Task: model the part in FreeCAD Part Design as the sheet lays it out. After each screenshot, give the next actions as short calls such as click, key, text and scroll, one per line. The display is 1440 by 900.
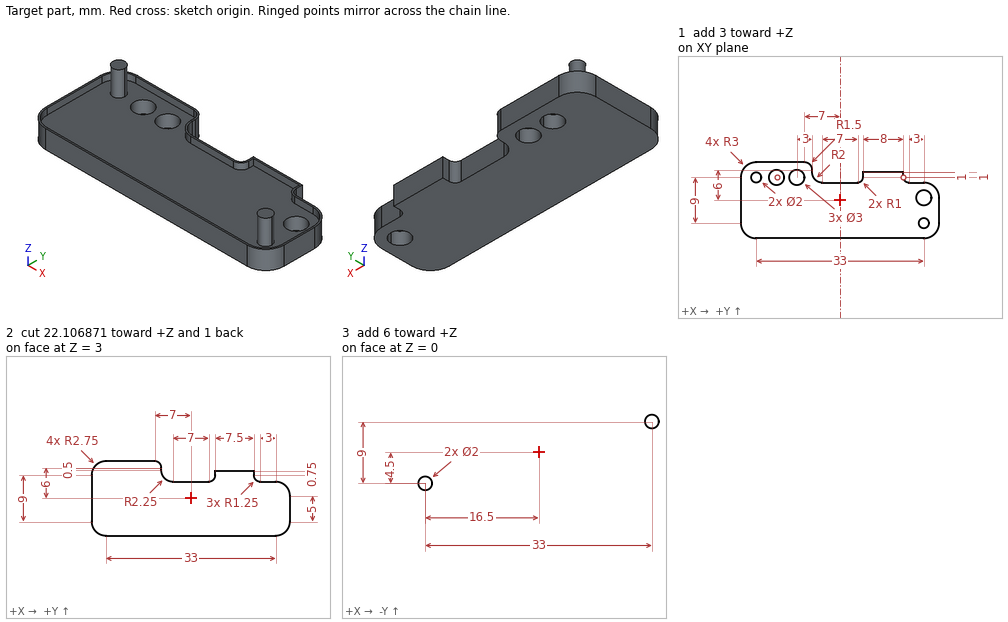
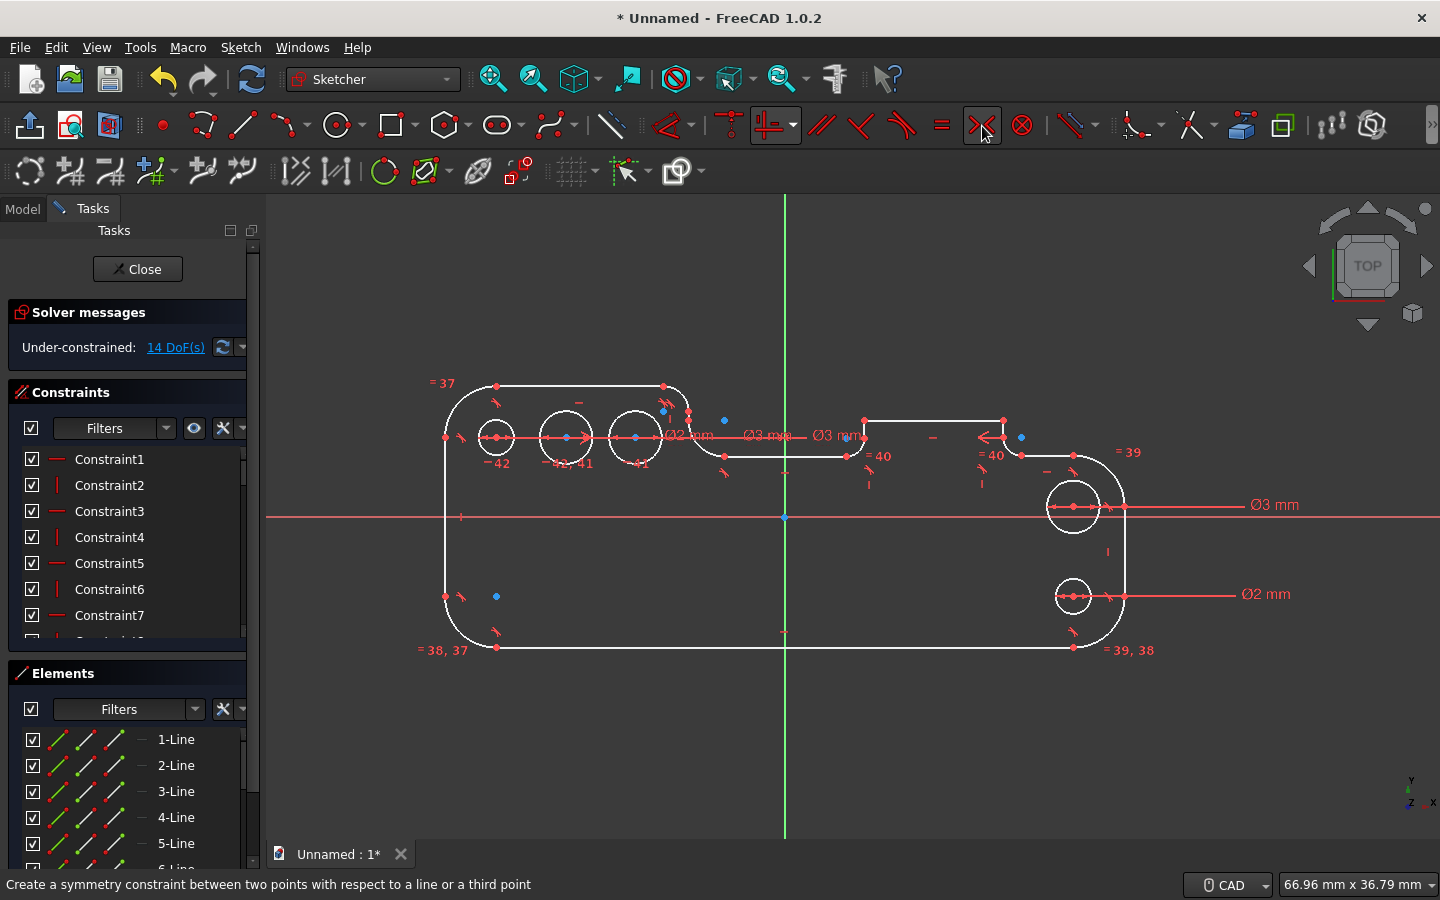
click(666, 126)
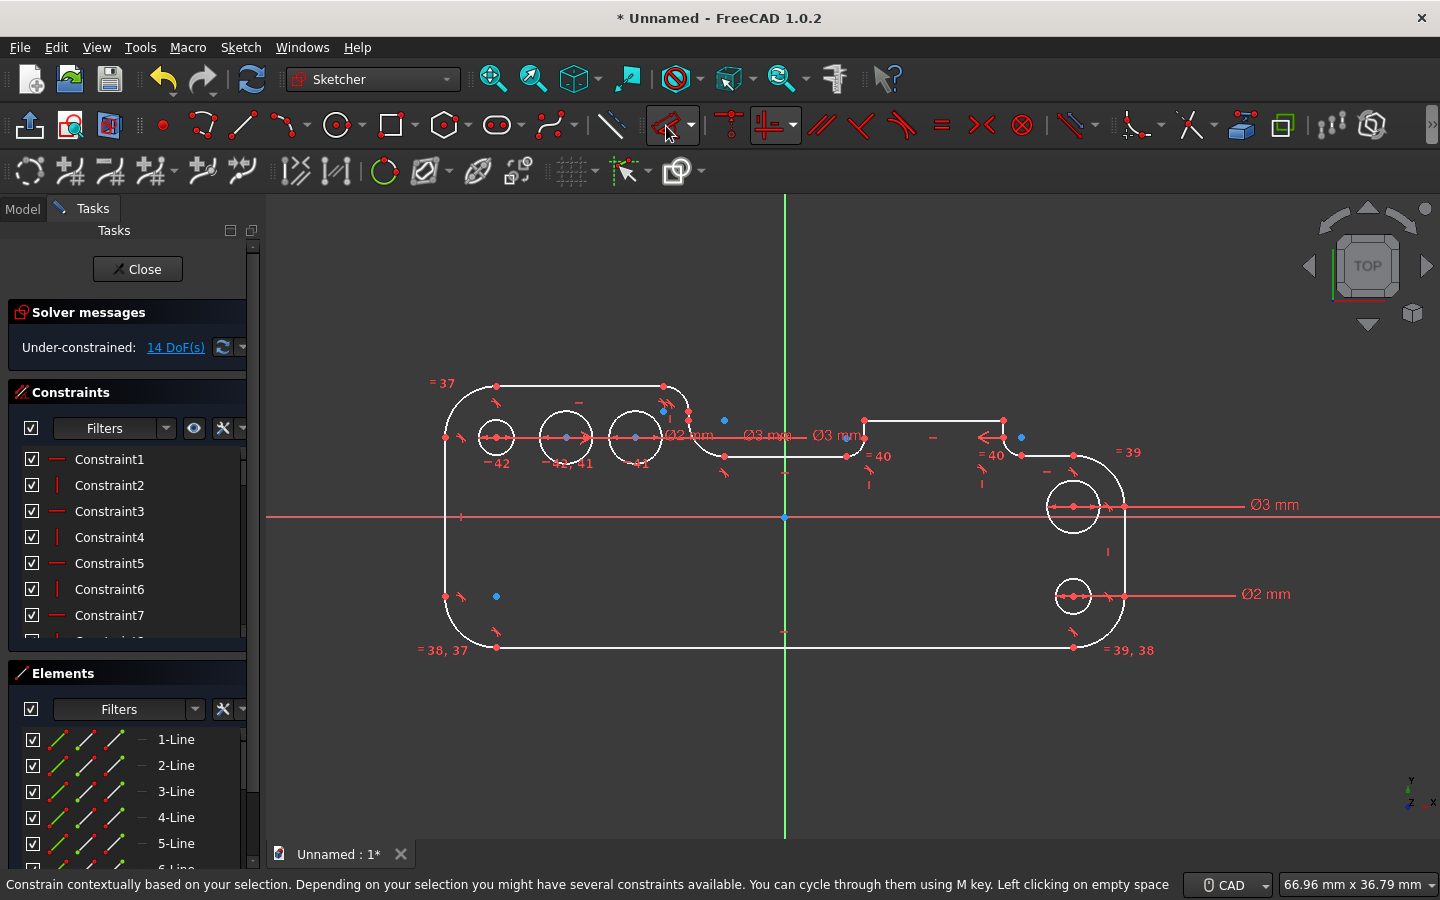
click(693, 437)
click(687, 477)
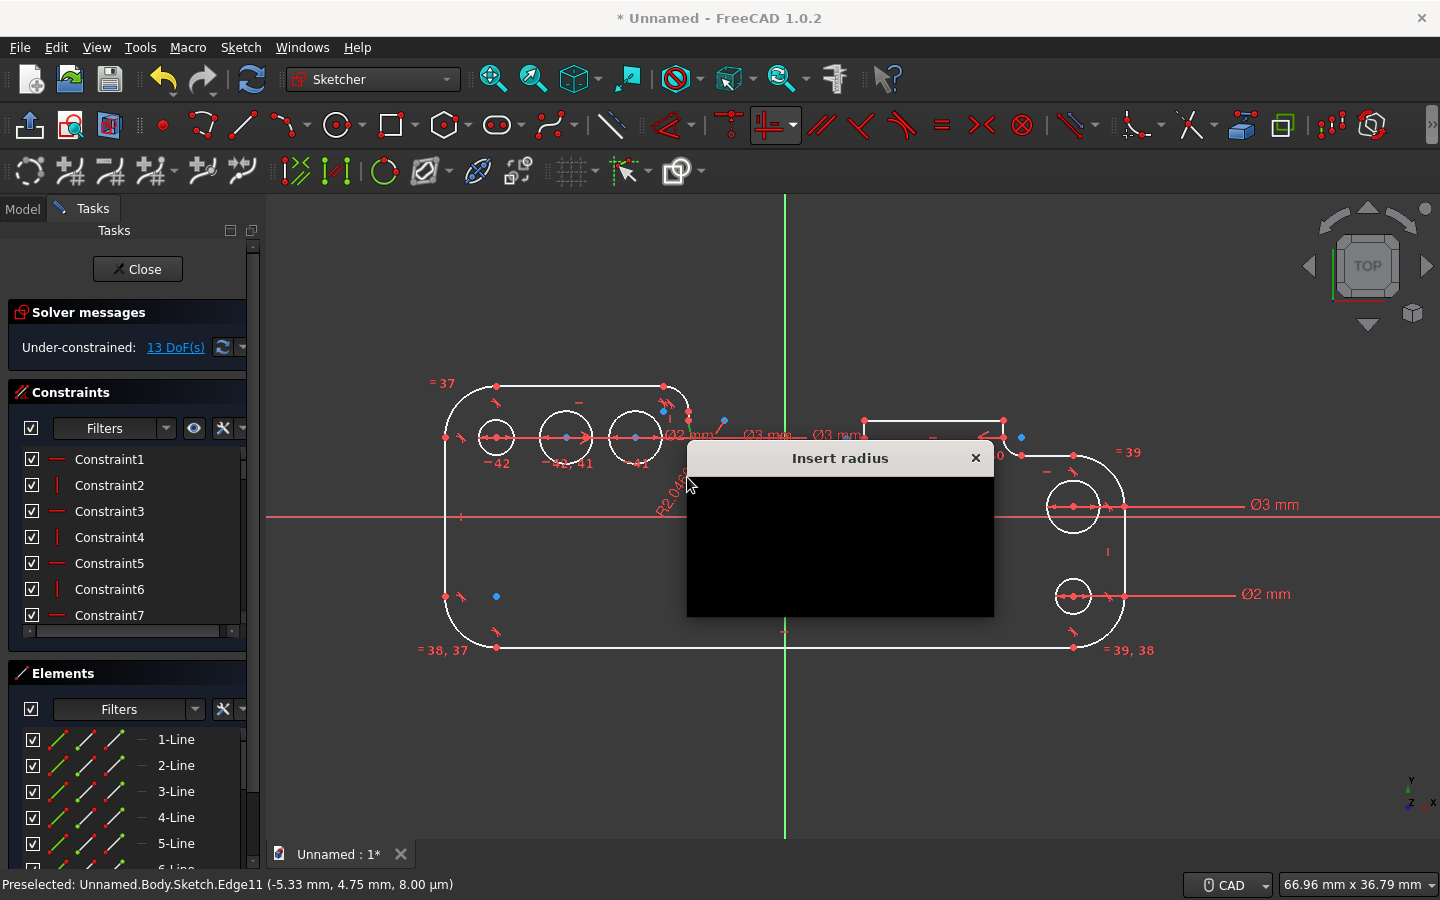
text(2)
key(Return)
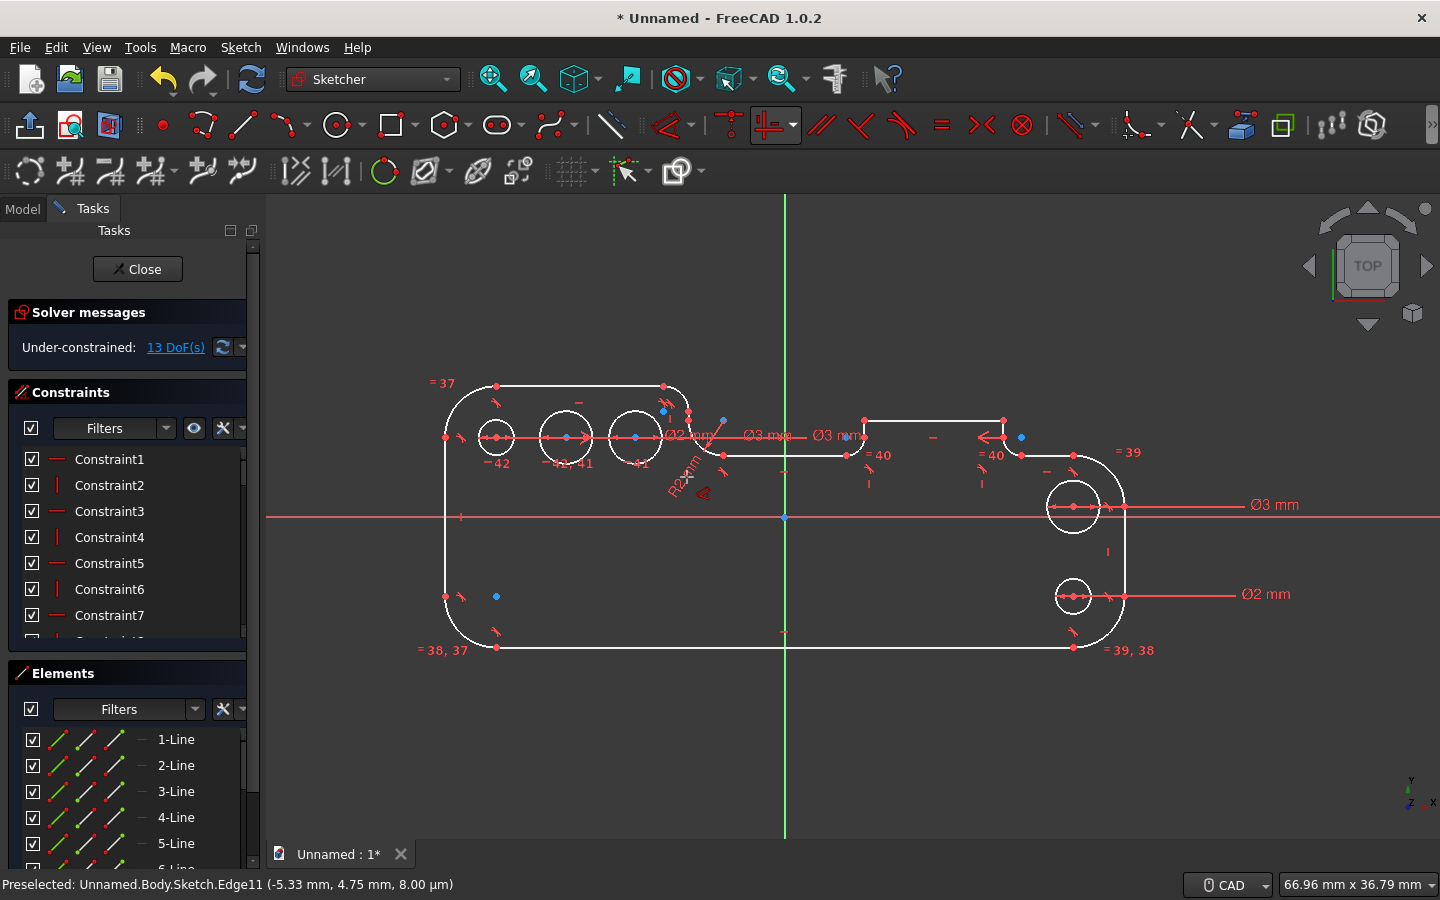
scroll(686, 400, up, 3)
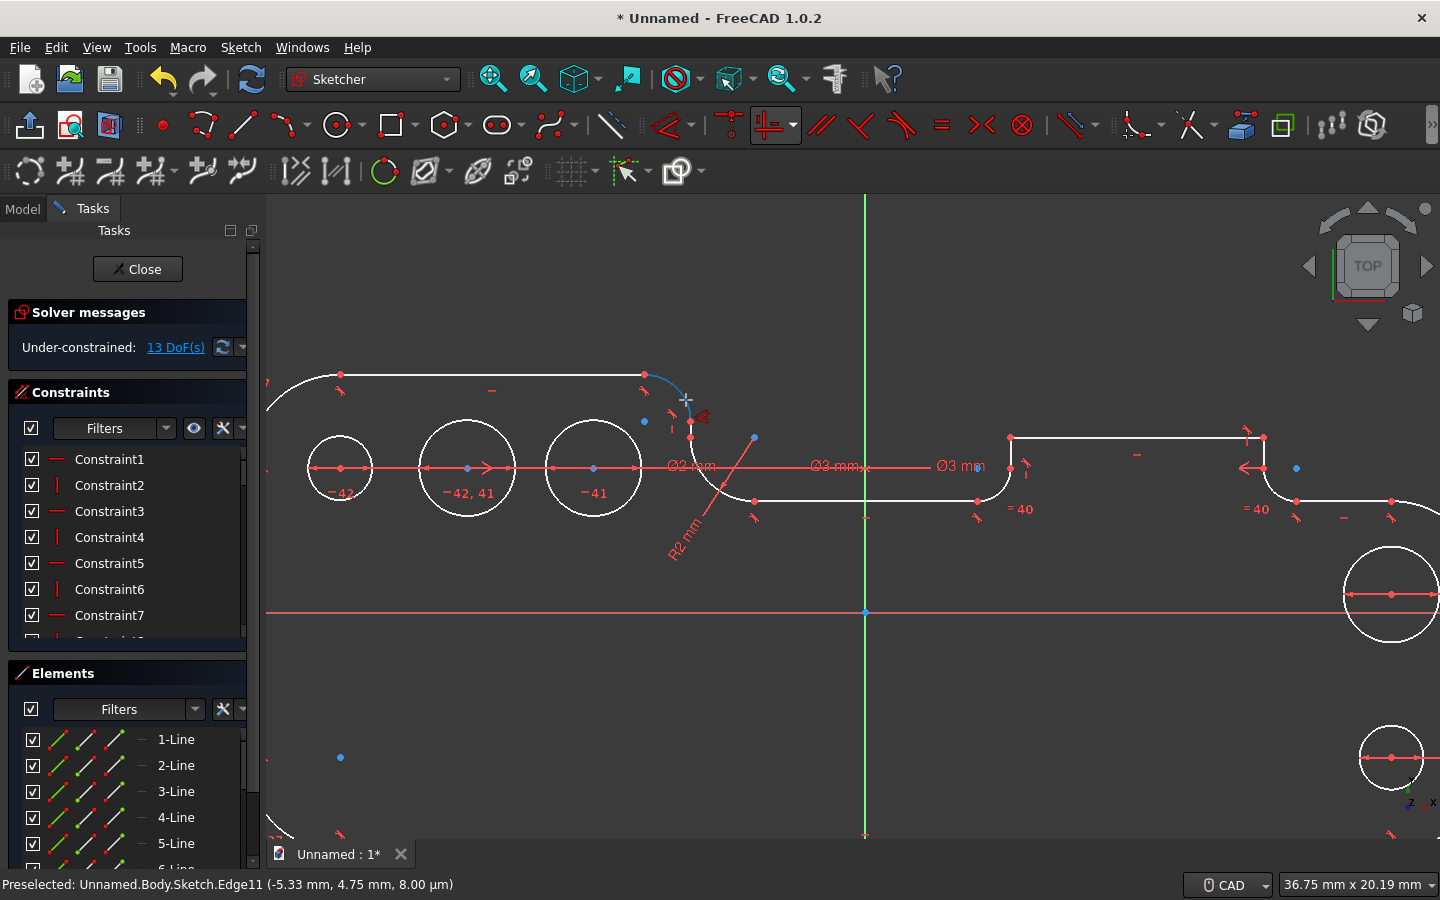
click(686, 400)
click(715, 386)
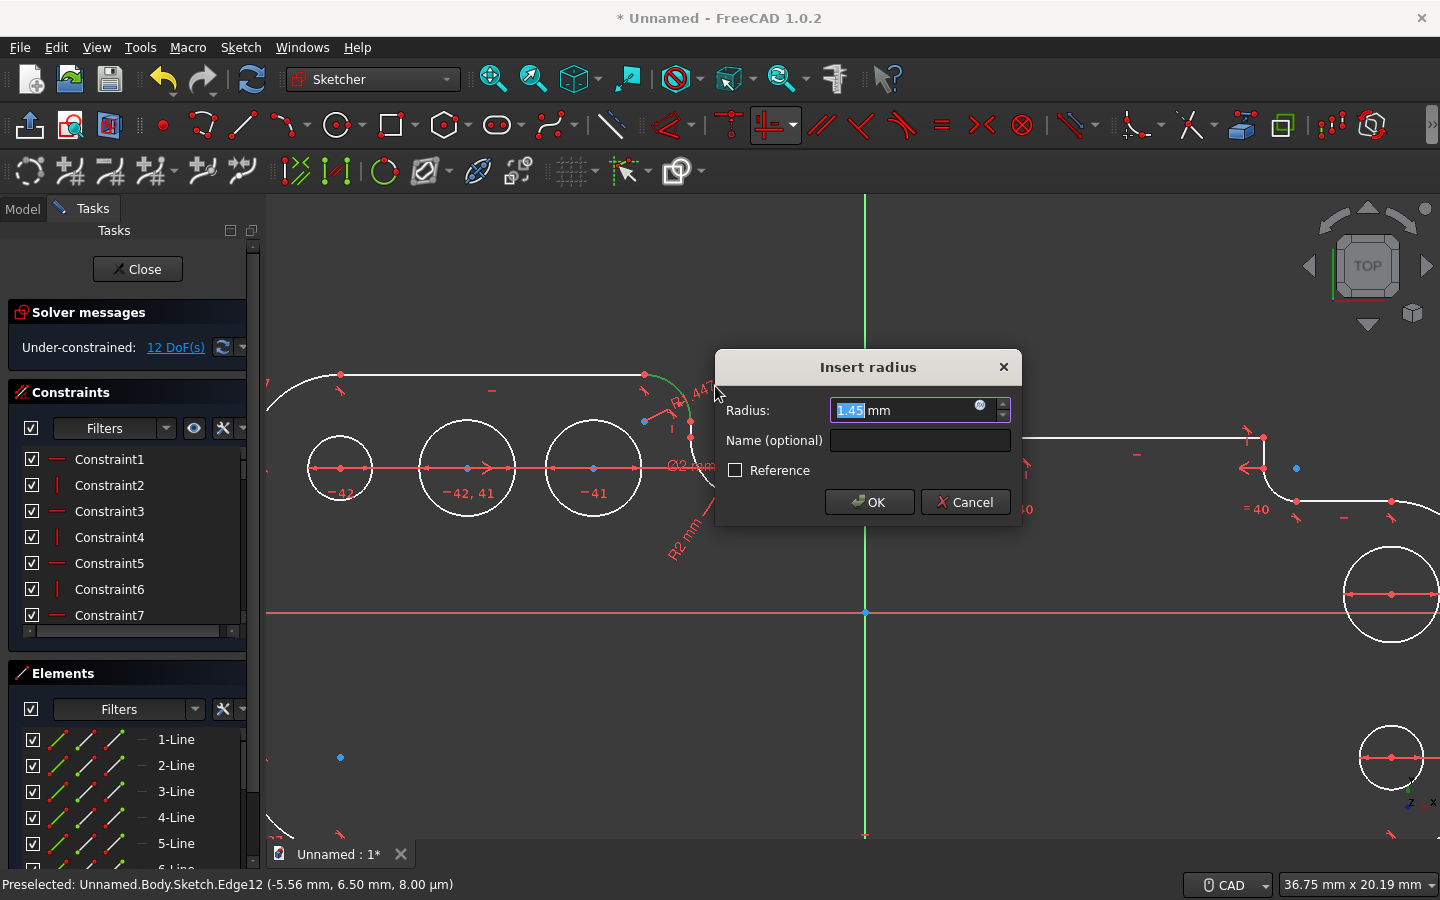
text(1.5)
key(Return)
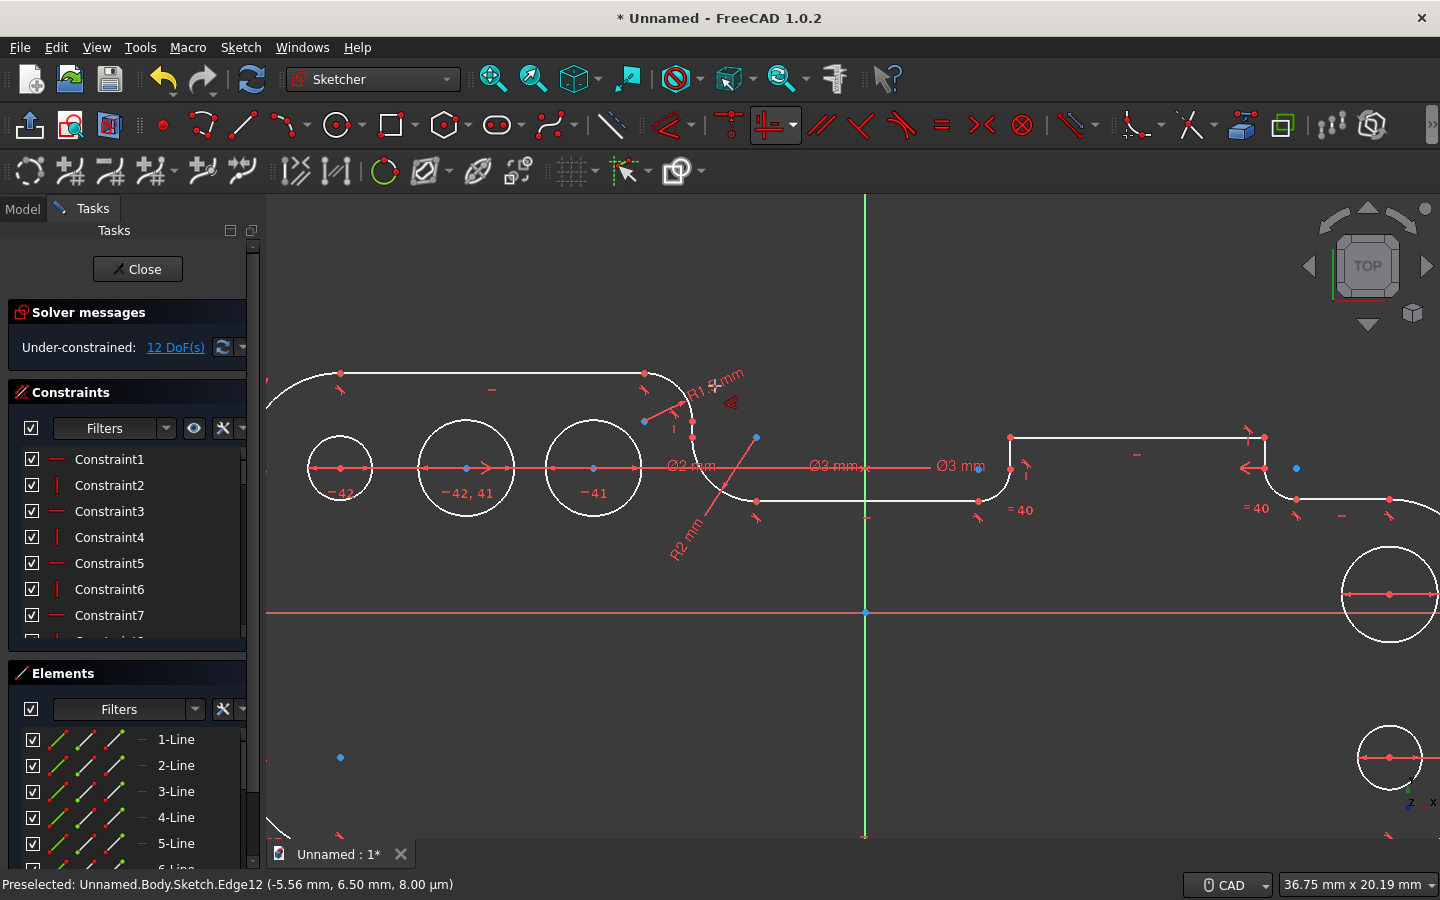
click(297, 383)
click(344, 341)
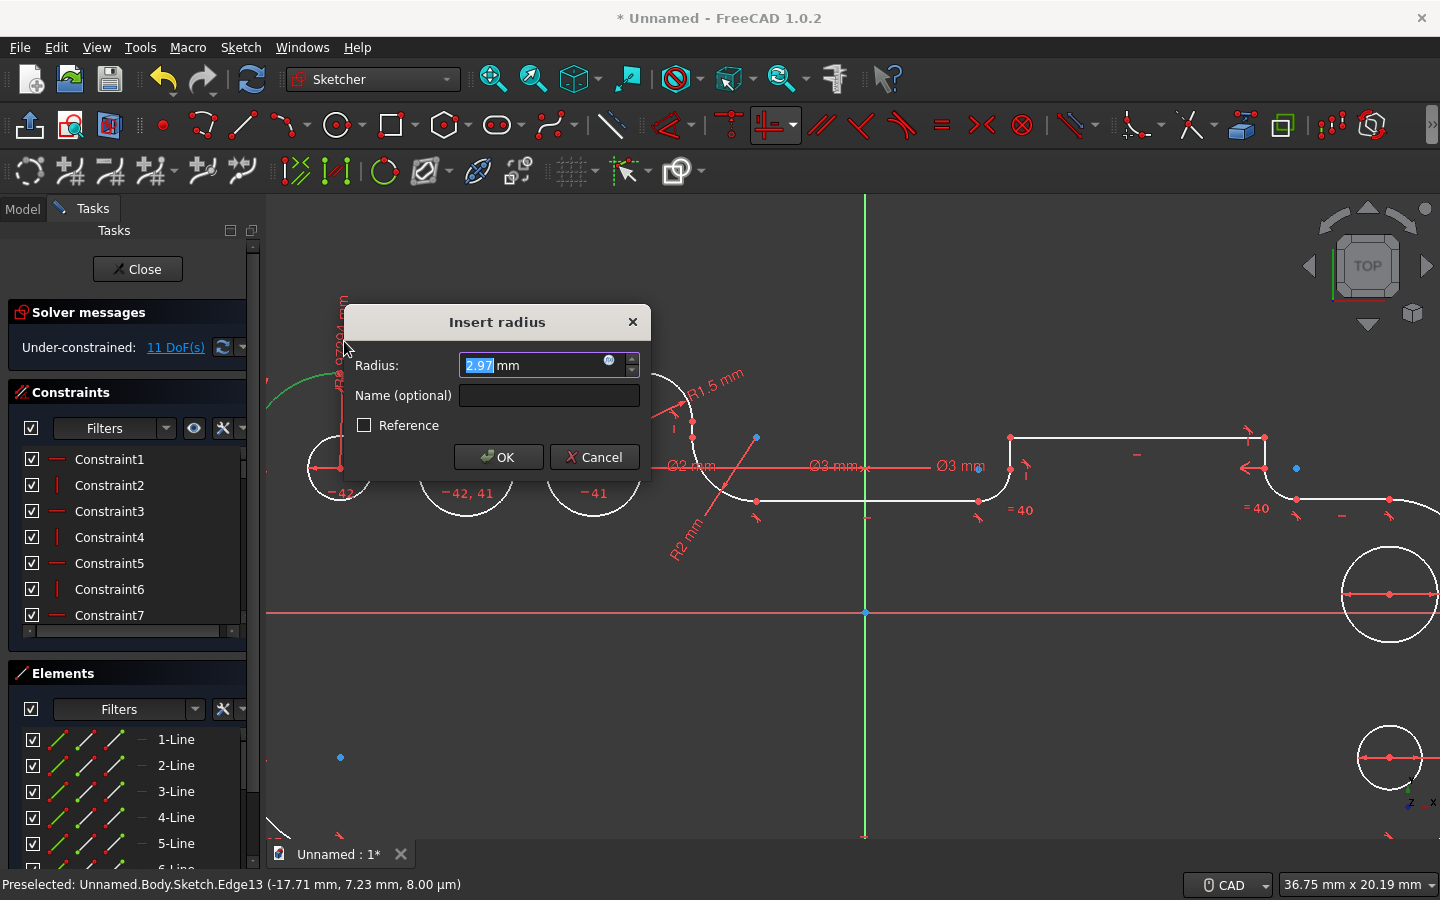
text(3)
key(Return)